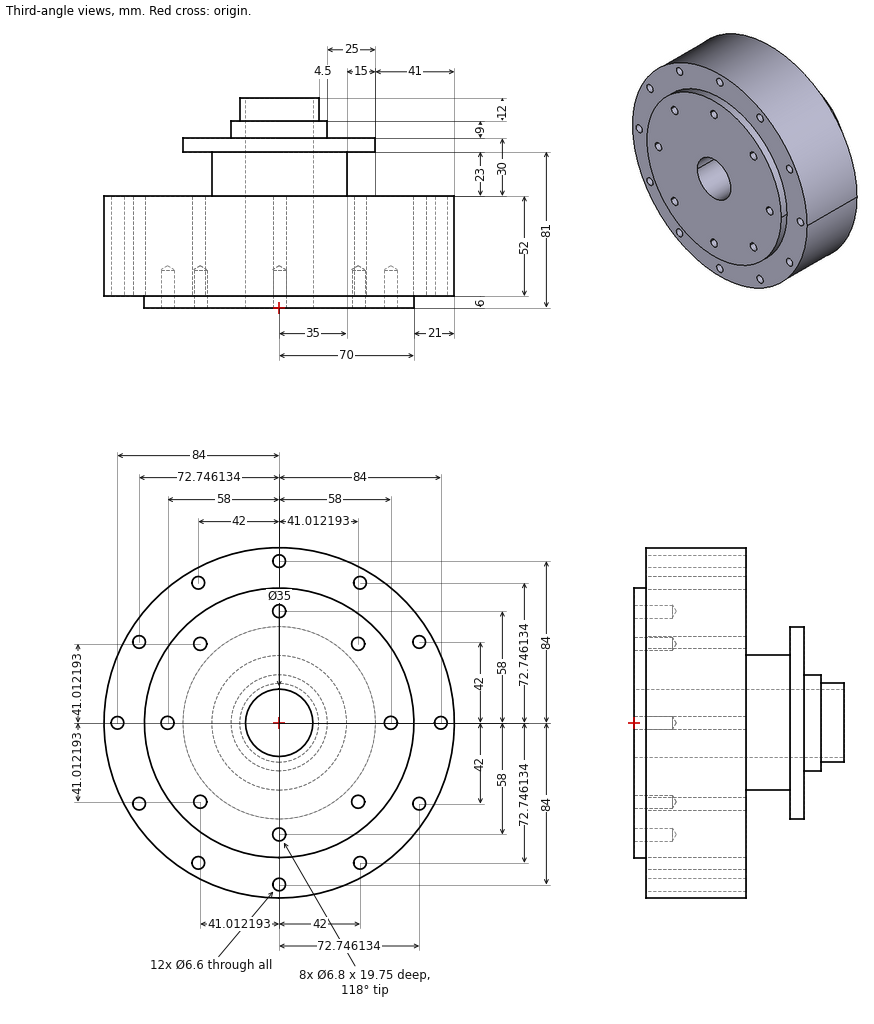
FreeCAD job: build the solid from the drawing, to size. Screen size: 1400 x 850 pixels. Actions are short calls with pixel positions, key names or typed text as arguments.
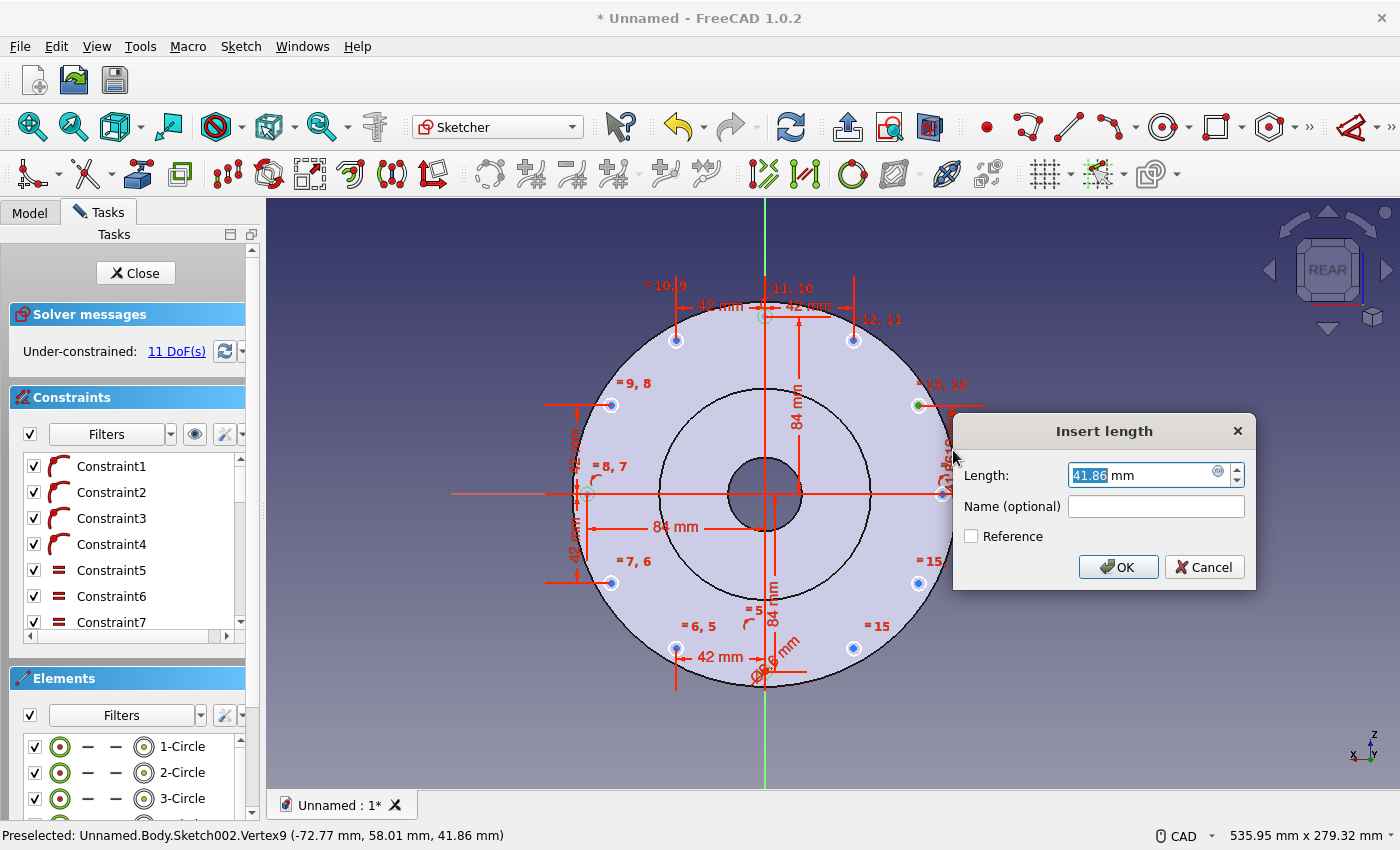
text(42)
key(Return)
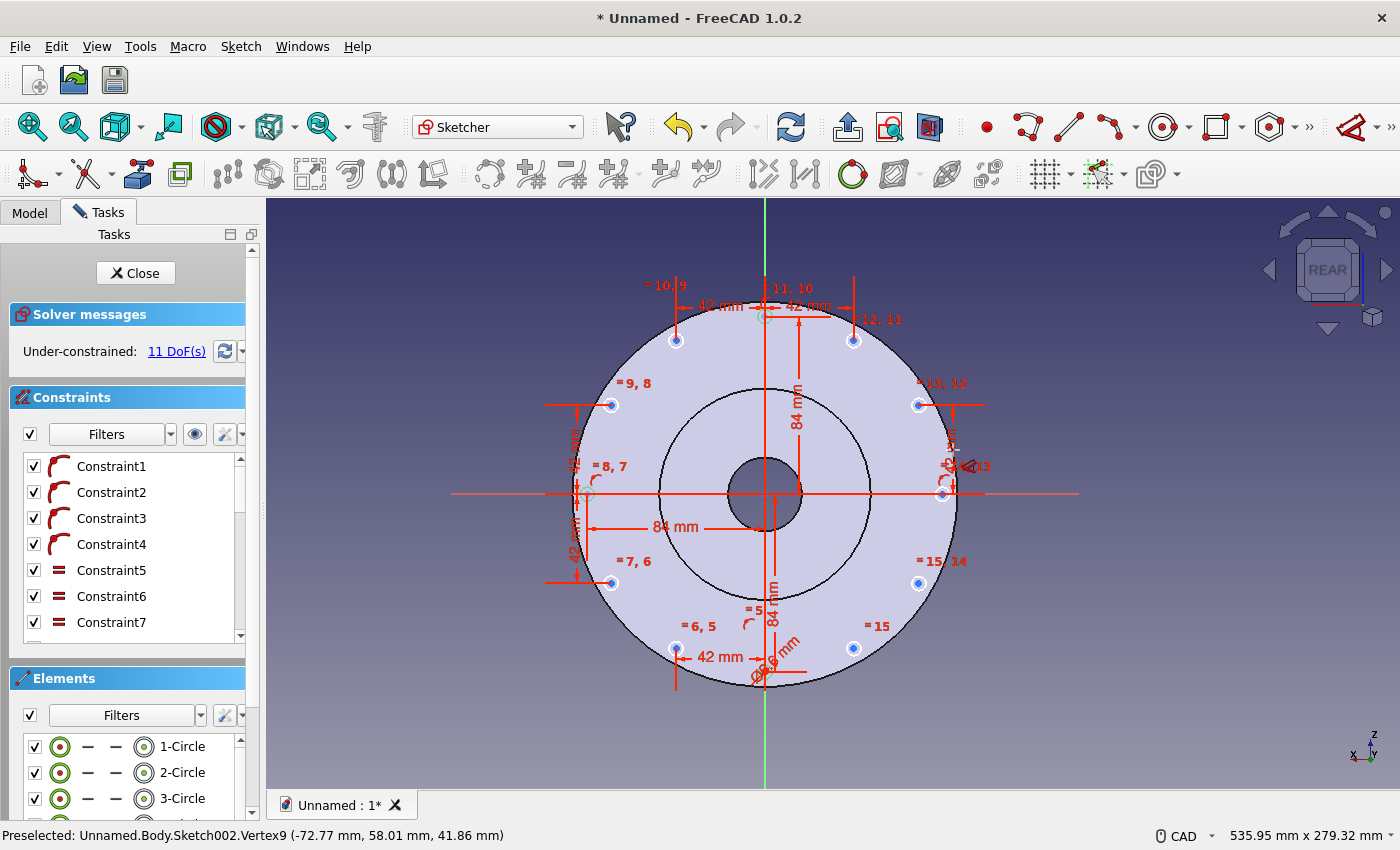
click(943, 494)
click(854, 528)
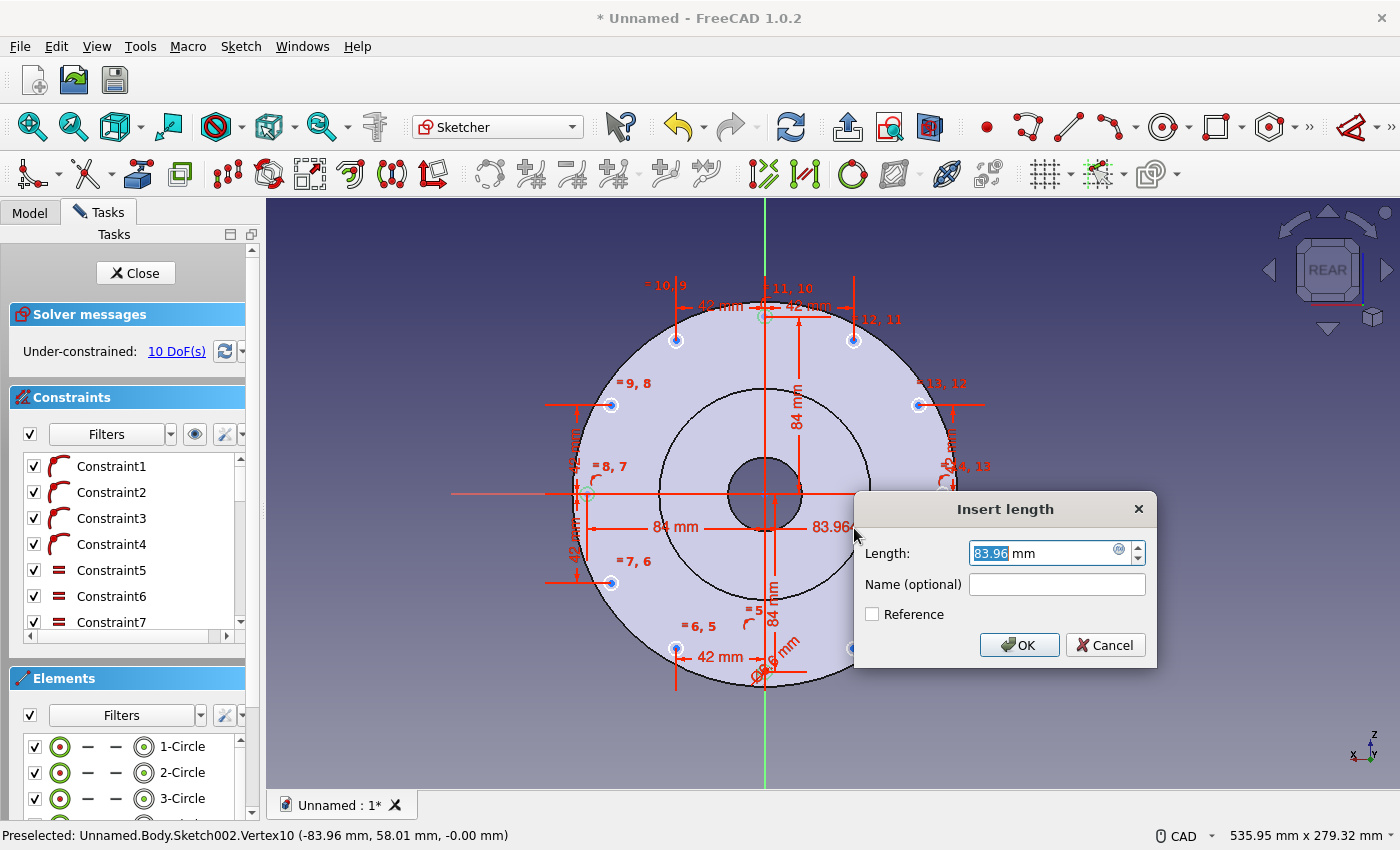
text(84)
key(Return)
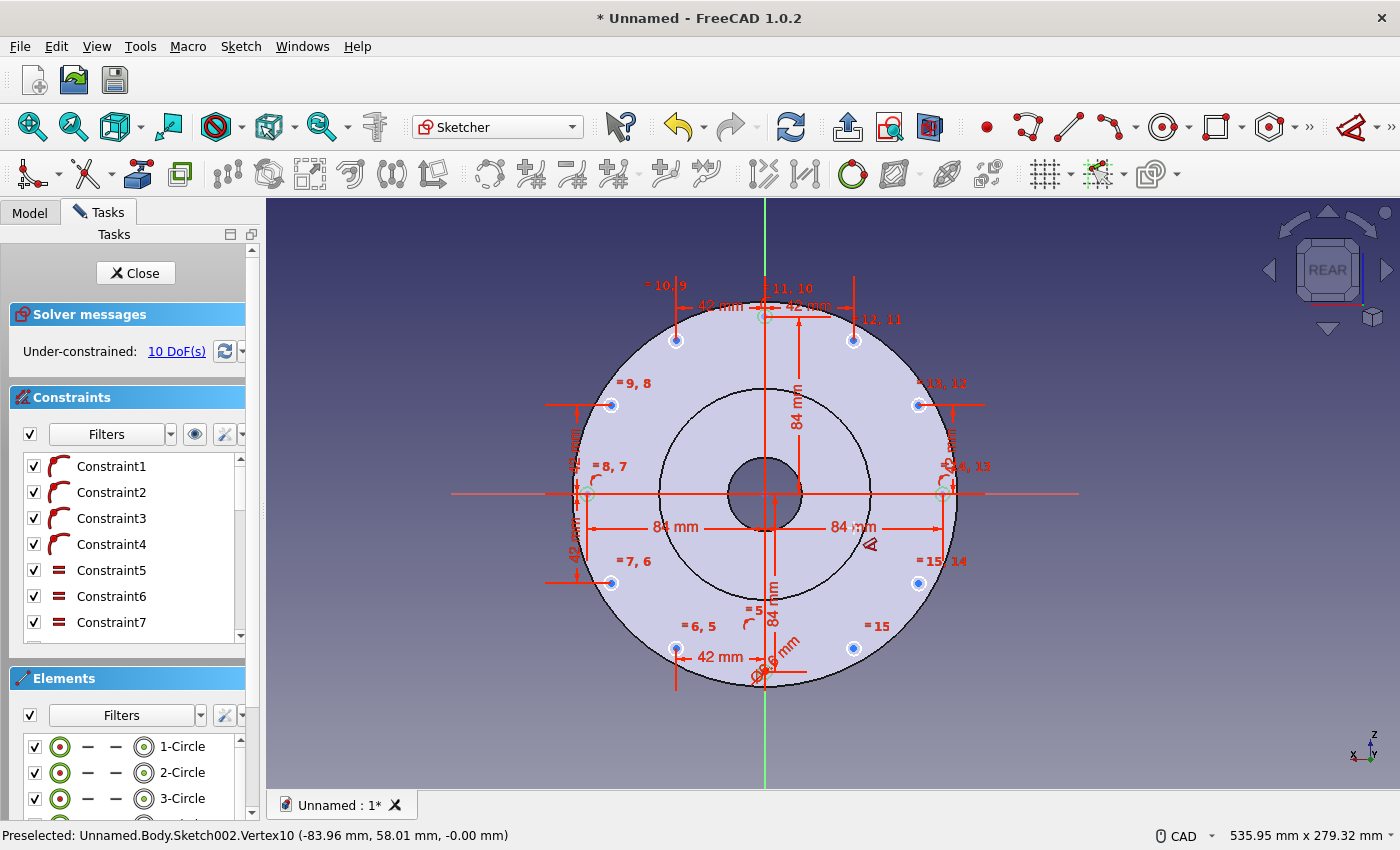
click(919, 584)
click(953, 539)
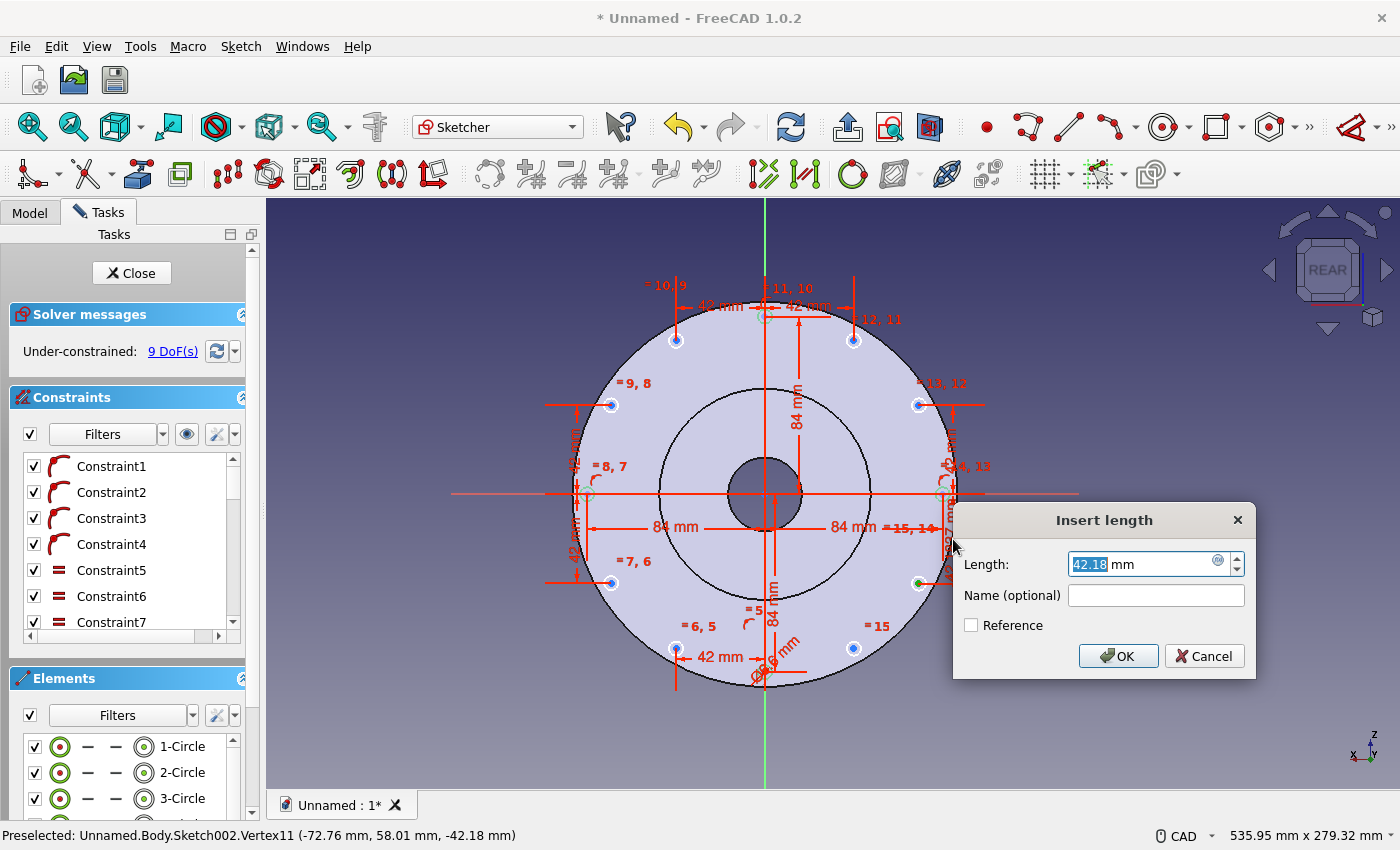
text(42)
key(Return)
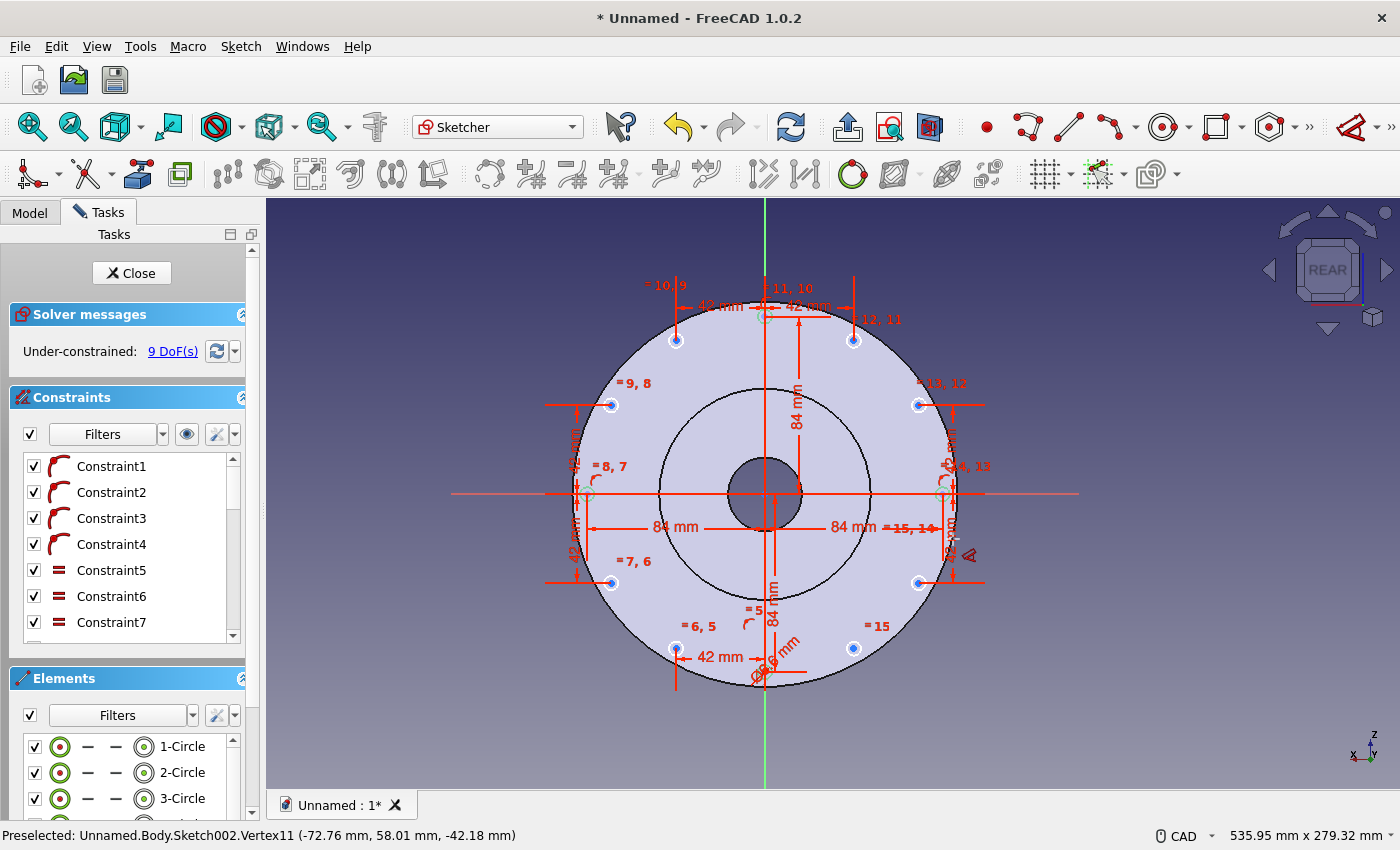
click(854, 649)
click(809, 683)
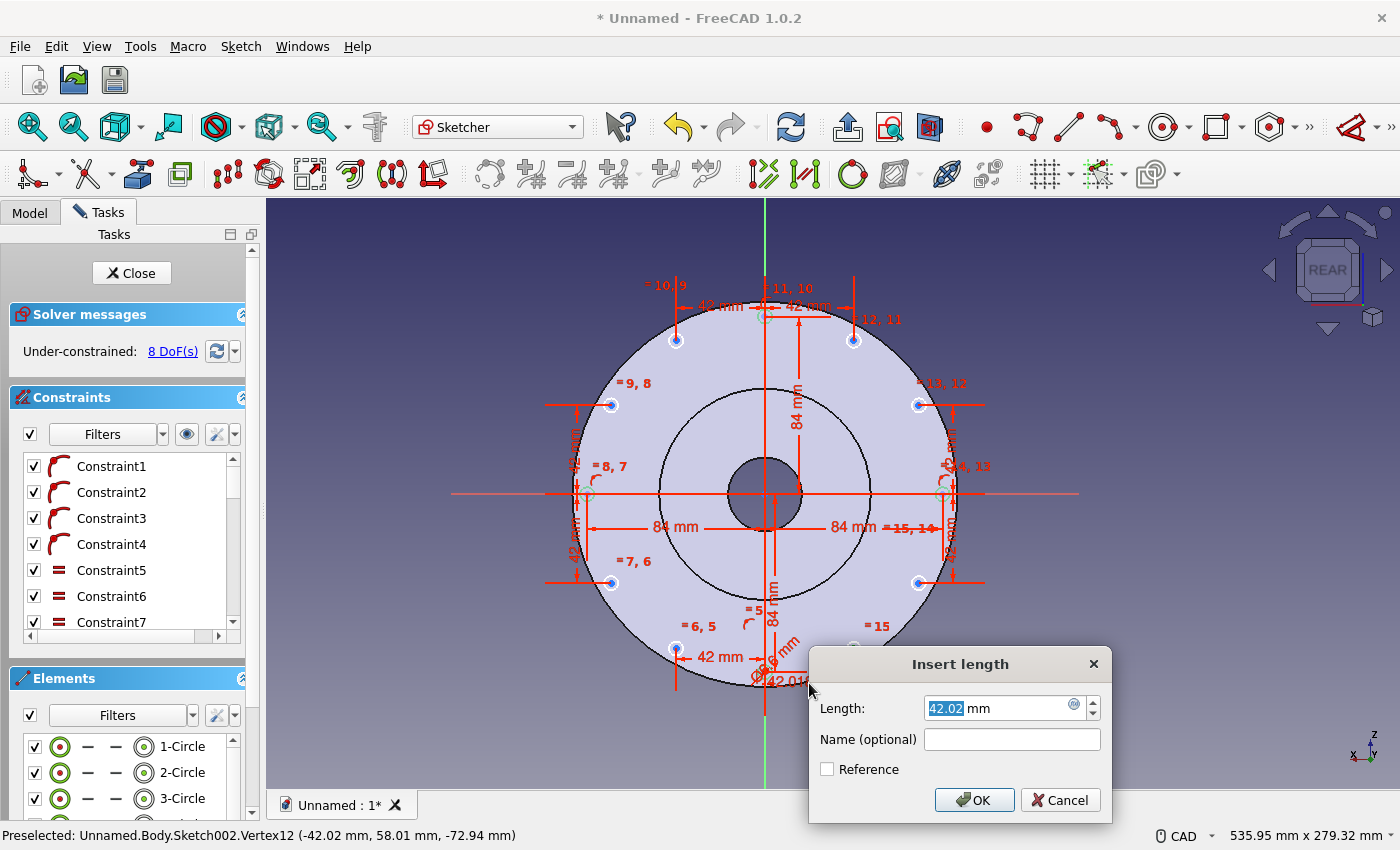
text(42)
key(Return)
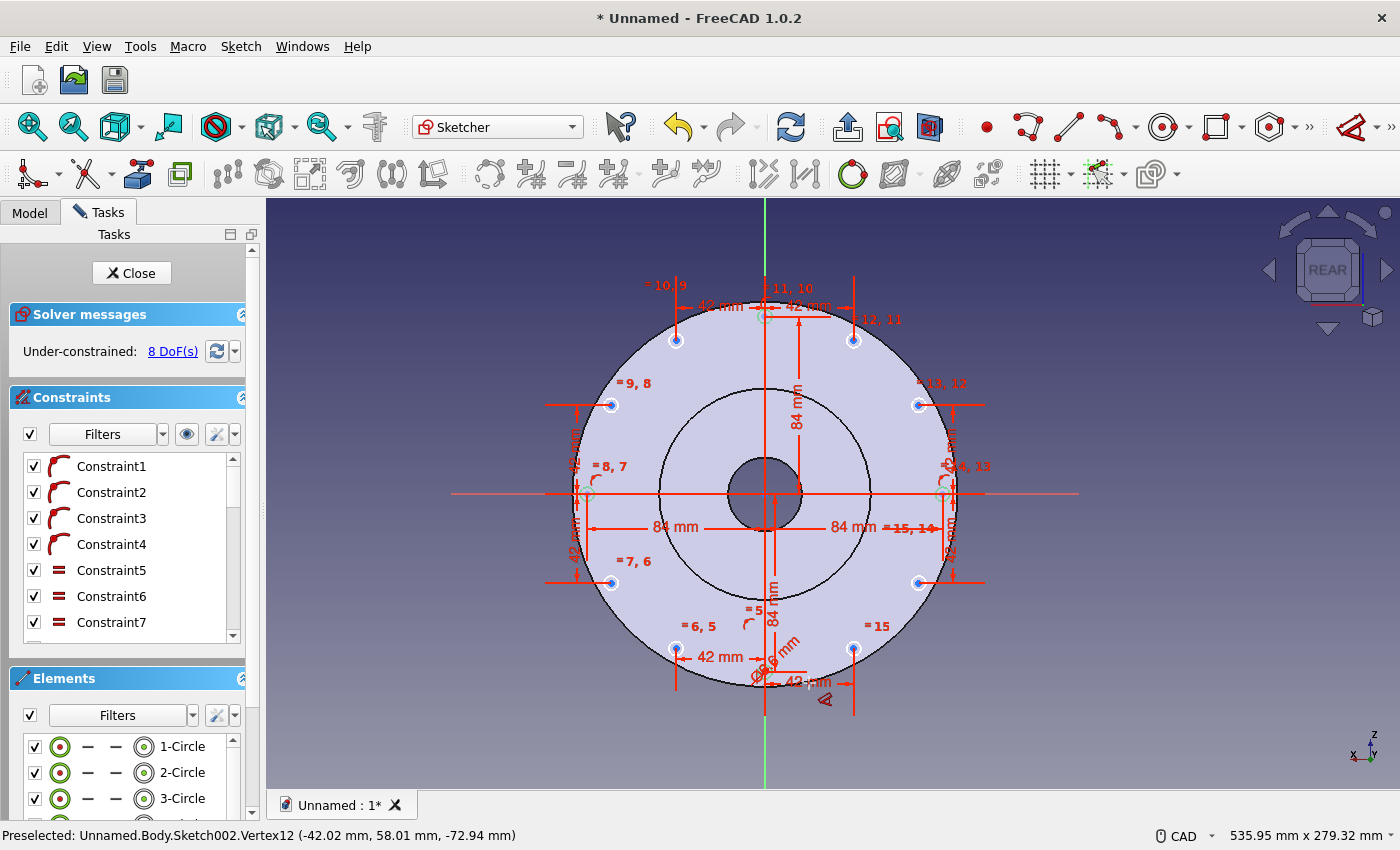
click(676, 649)
click(642, 571)